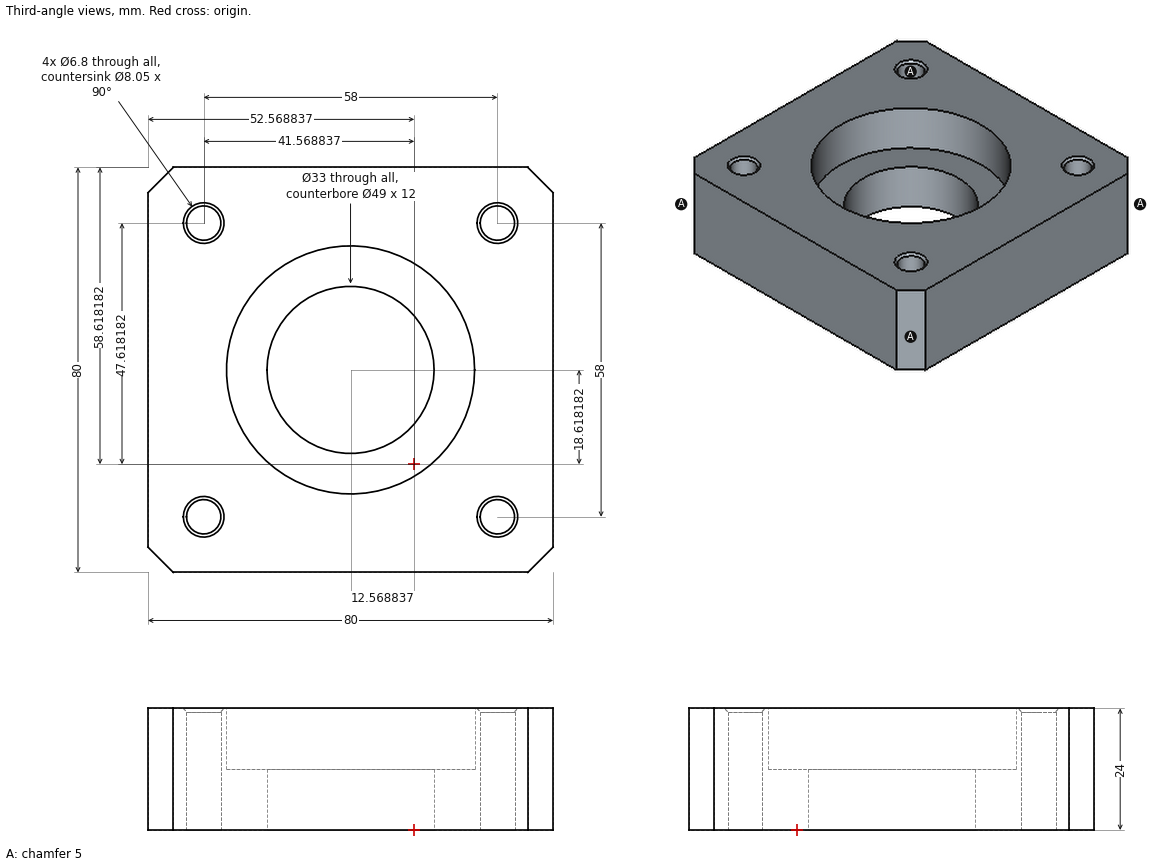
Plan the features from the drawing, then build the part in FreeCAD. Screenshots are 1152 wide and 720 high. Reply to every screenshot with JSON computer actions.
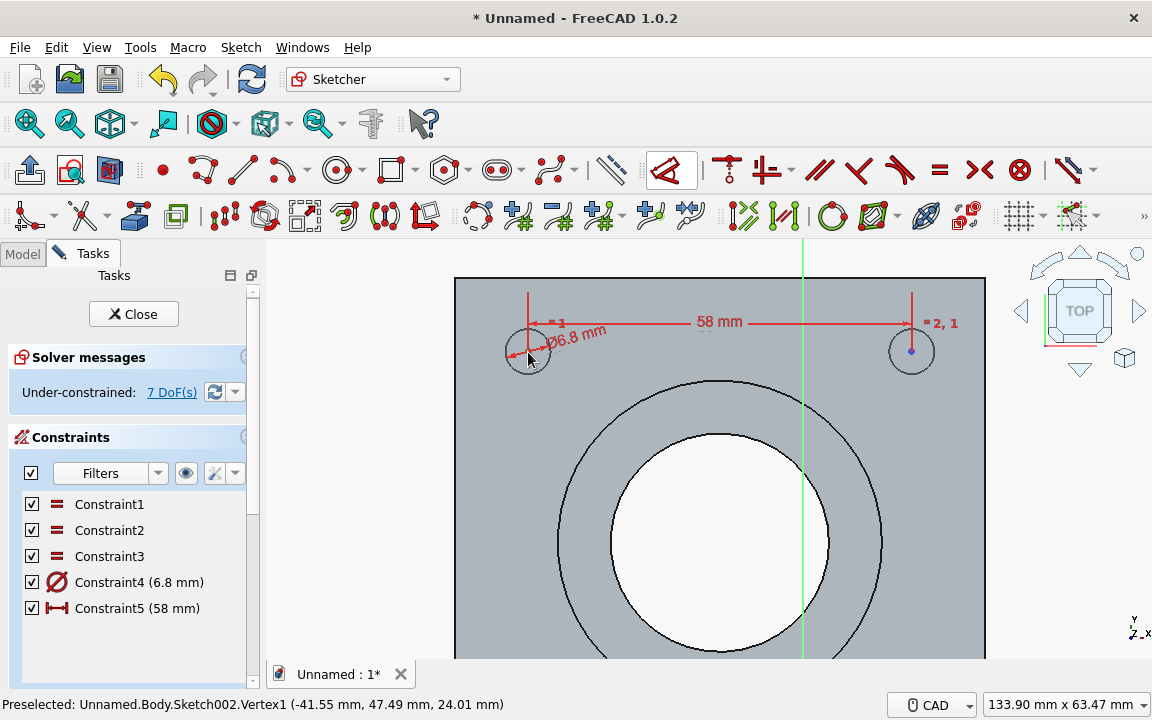
{"action": "scroll", "coordinate": [544, 335], "scroll_direction": "down", "scroll_amount": 3}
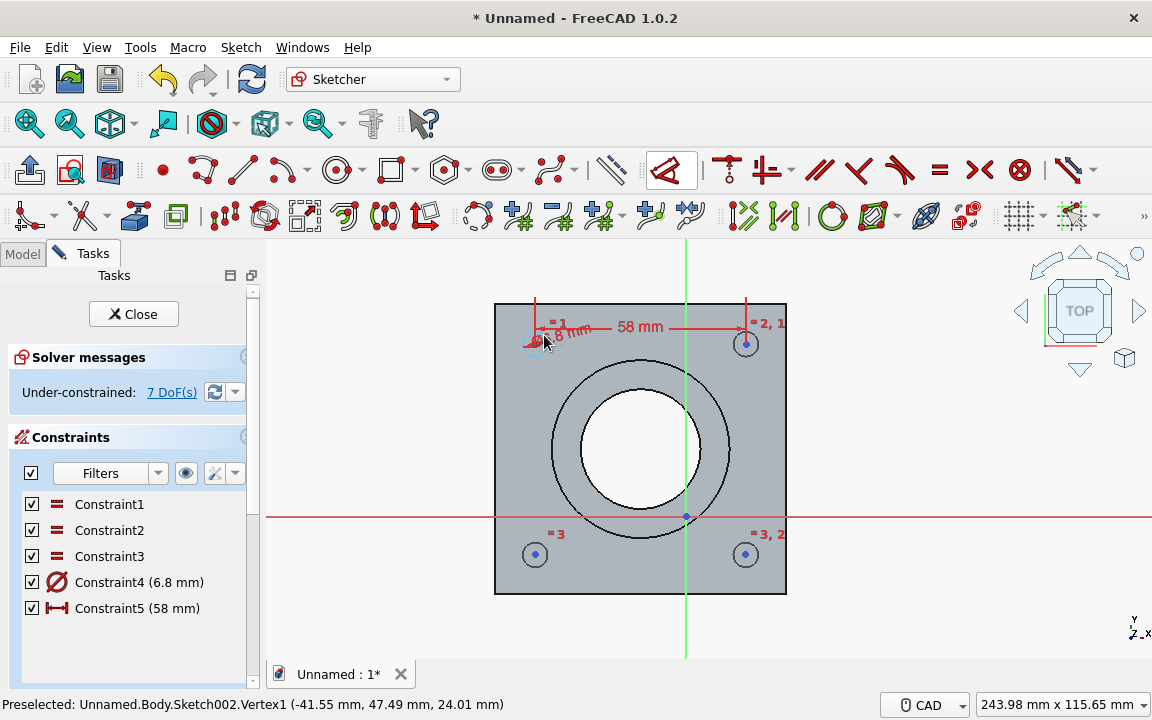
{"action": "left_click", "coordinate": [746, 555]}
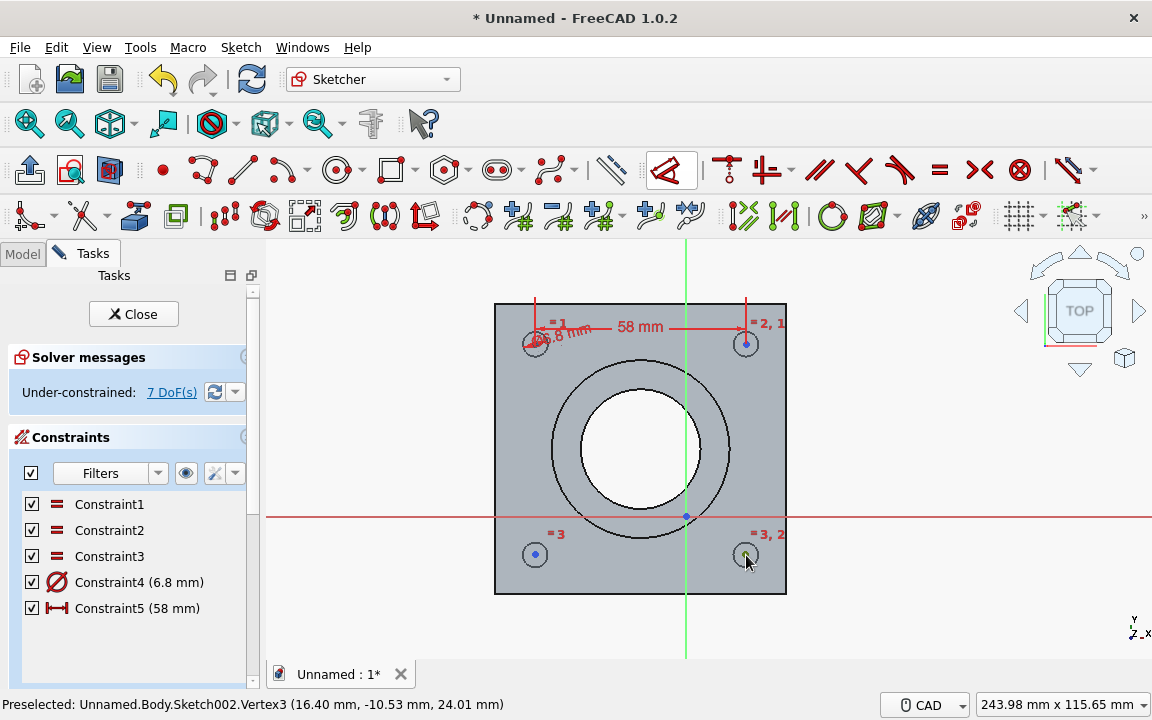
{"action": "key", "text": "l"}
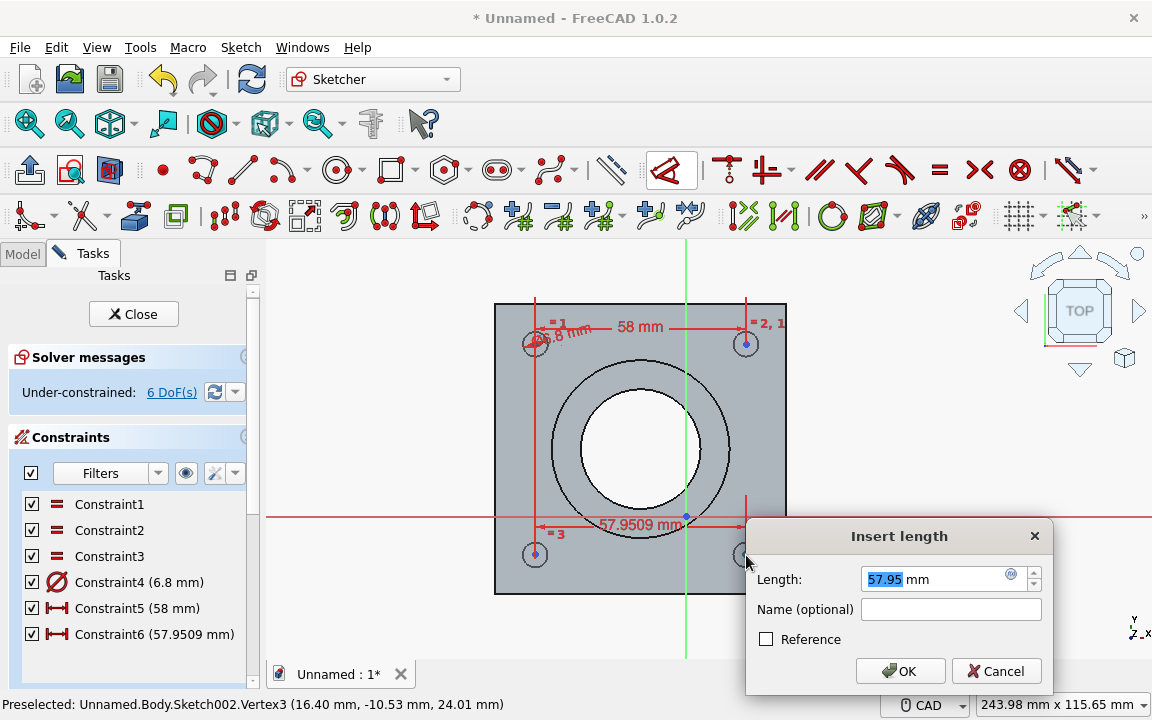
{"action": "type", "text": "58"}
{"action": "key", "text": "Return"}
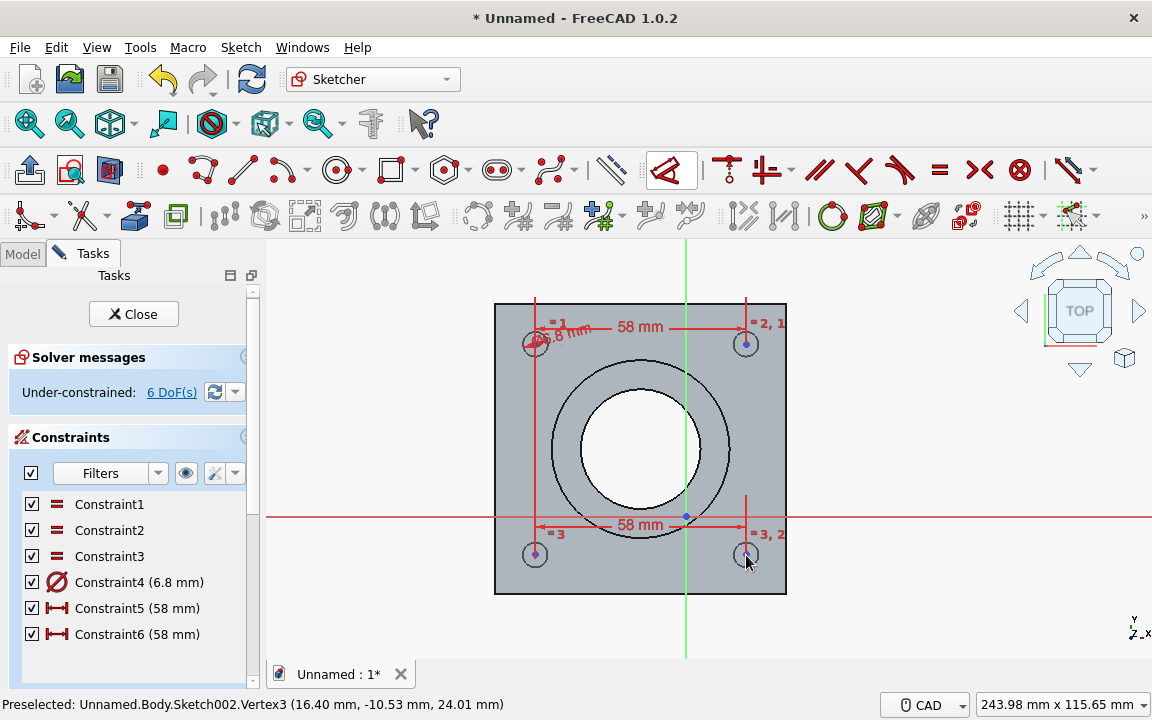
{"action": "left_click", "coordinate": [746, 344]}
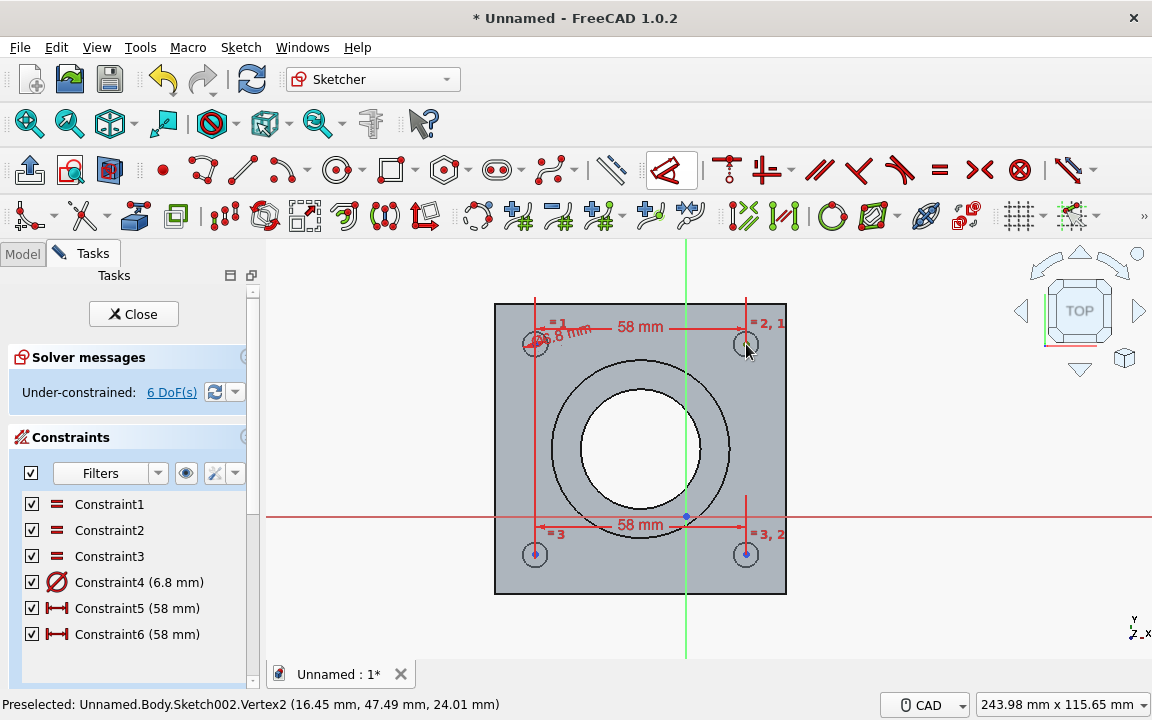
{"action": "left_click", "coordinate": [746, 555]}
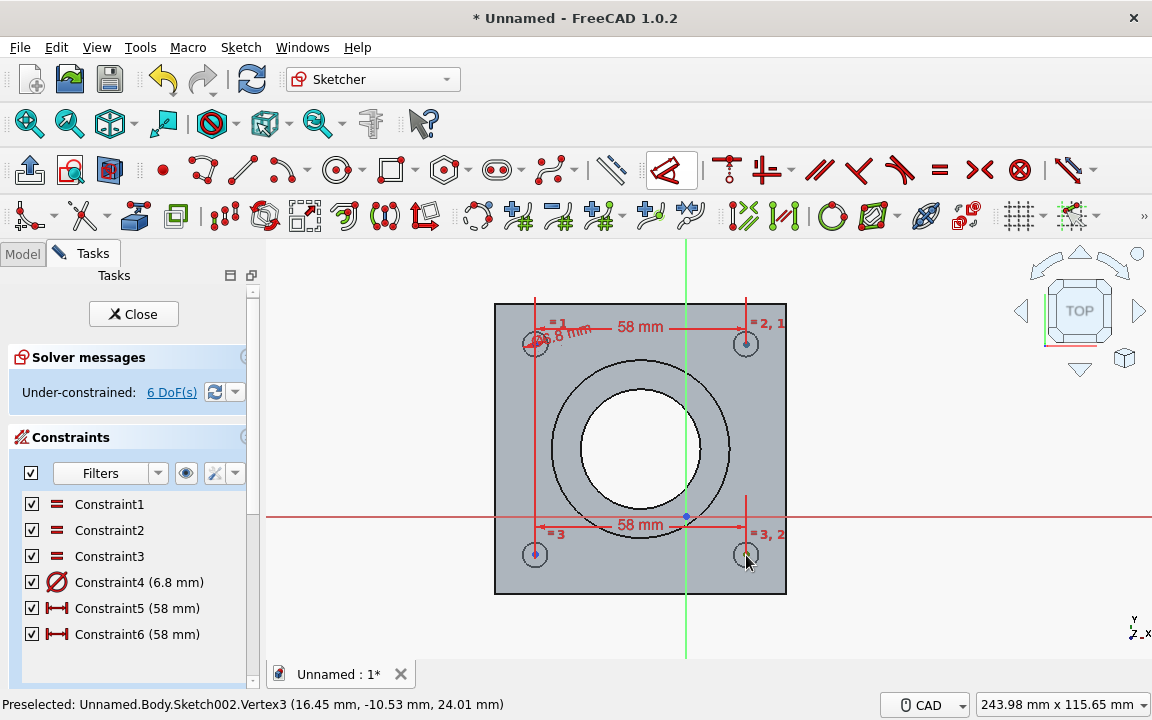
{"action": "left_click", "coordinate": [692, 170]}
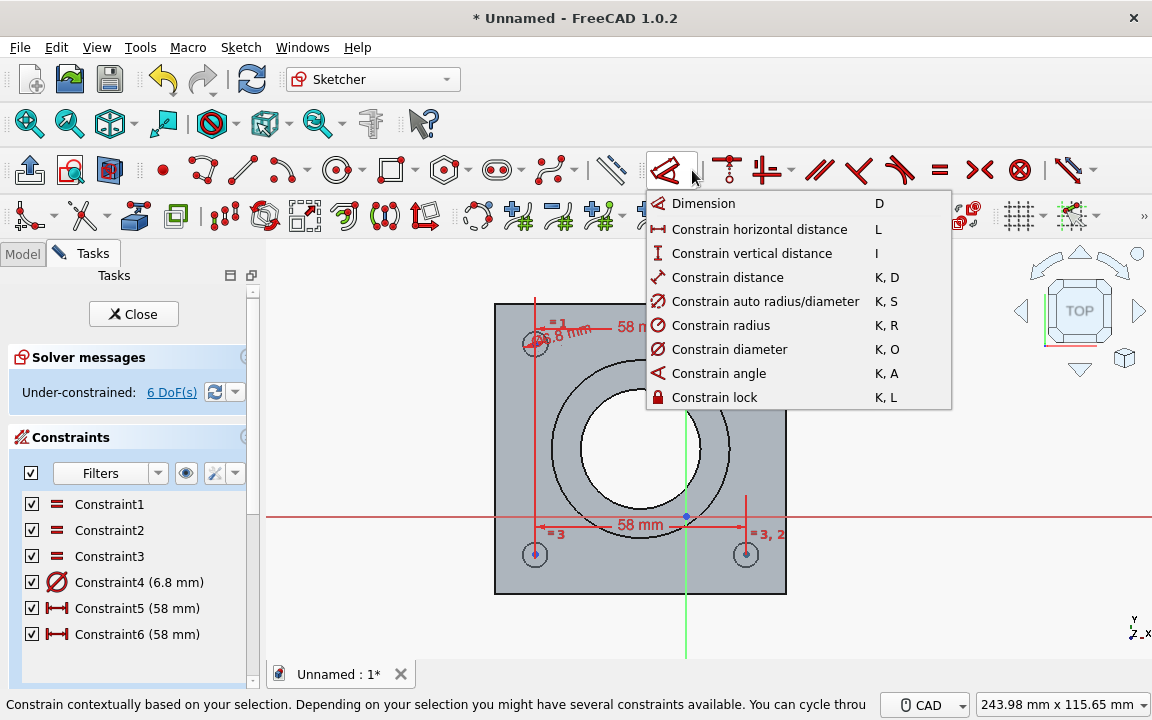
{"action": "left_click", "coordinate": [799, 253]}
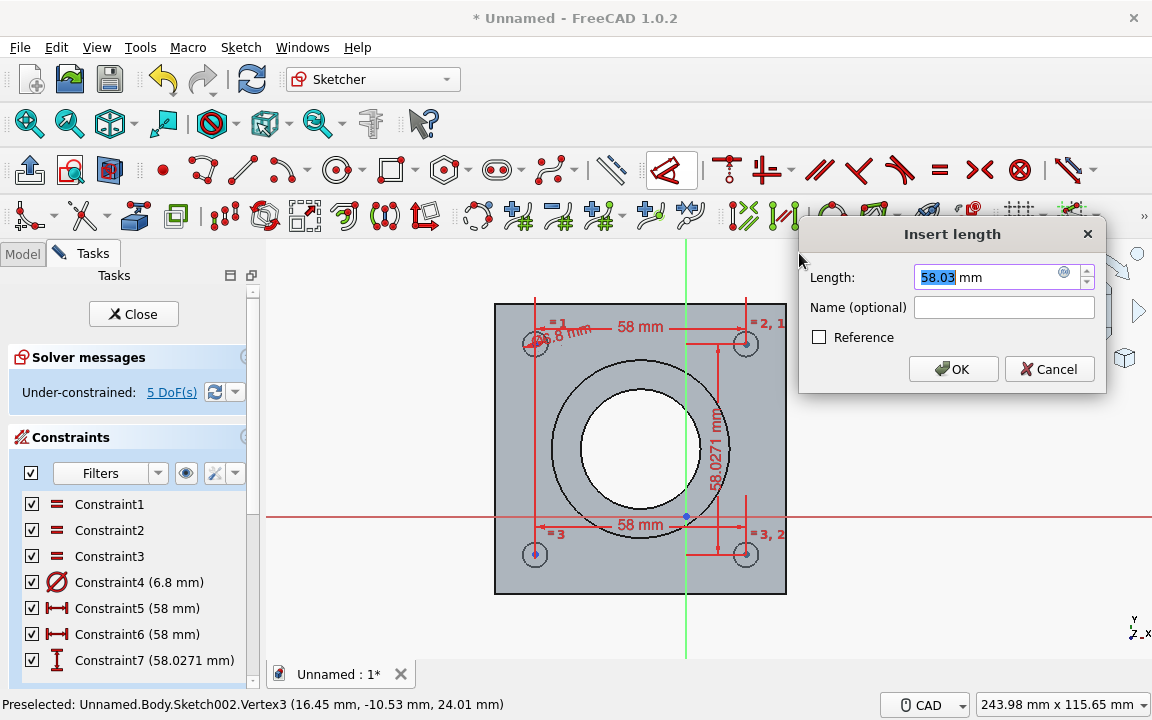
{"action": "type", "text": "58"}
{"action": "key", "text": "Return"}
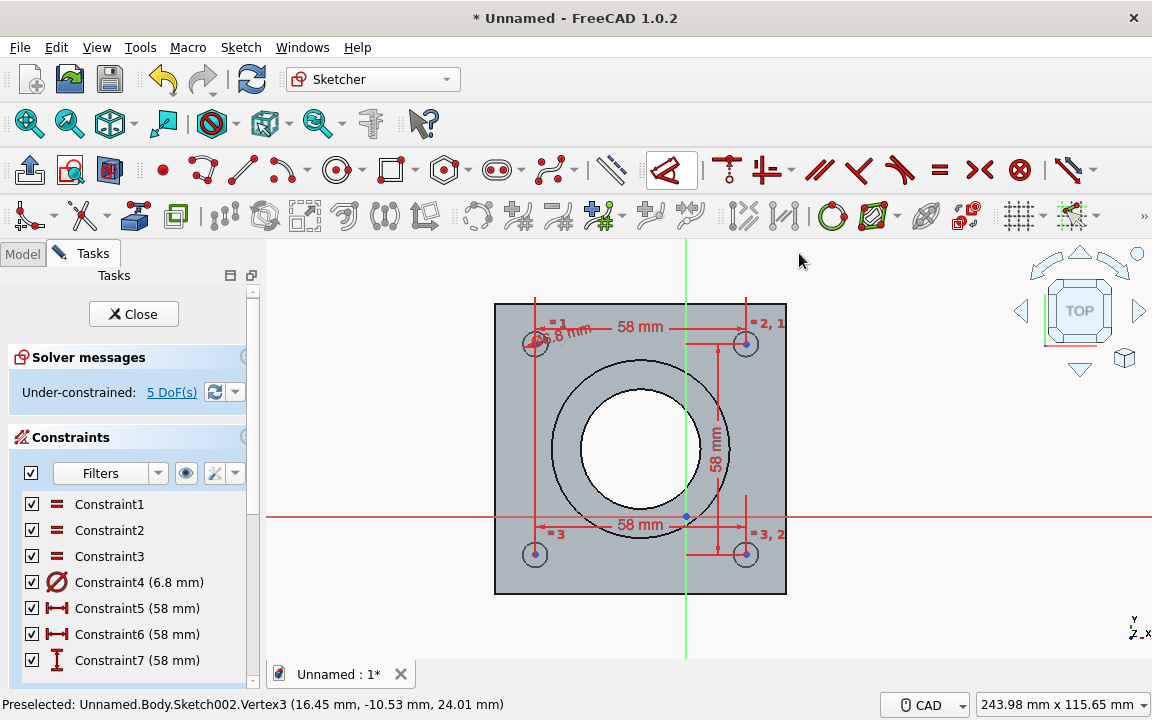
{"action": "left_click", "coordinate": [535, 344]}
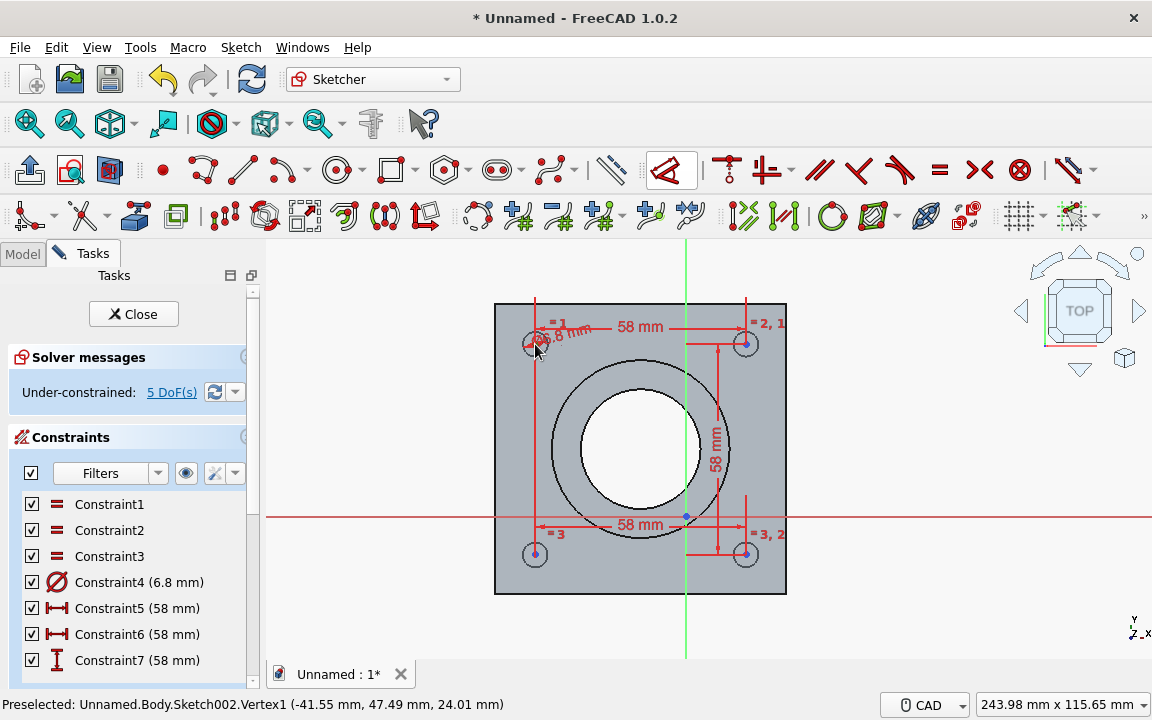
{"action": "left_click", "coordinate": [746, 555]}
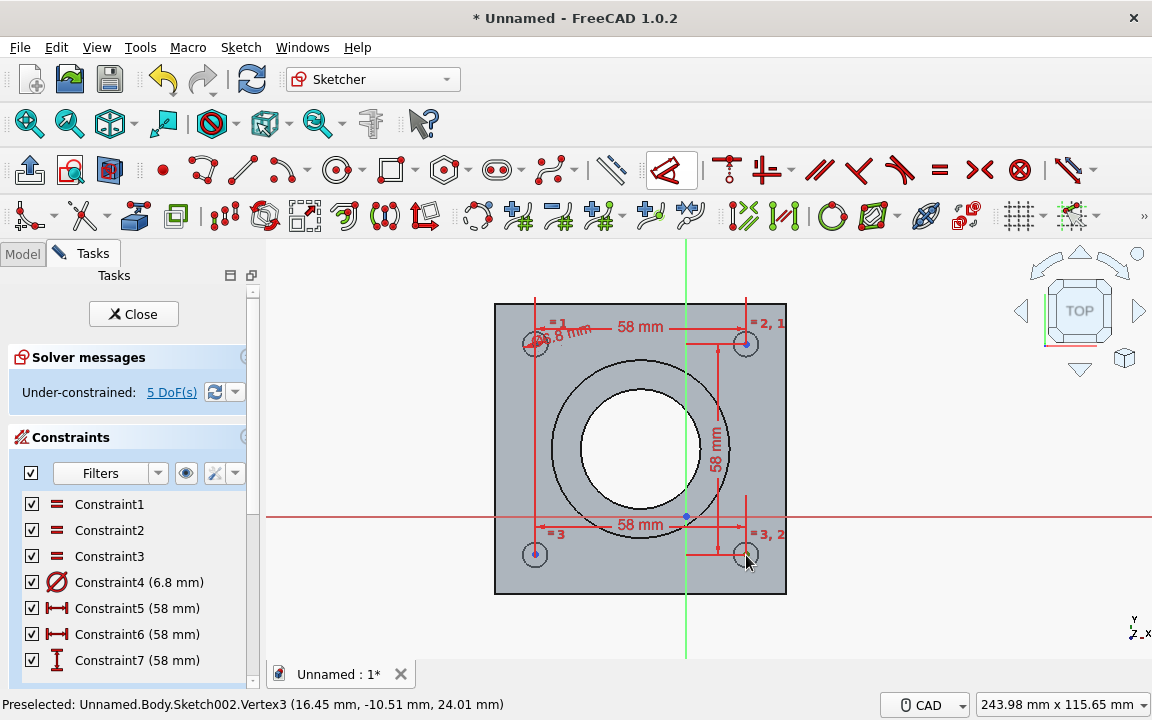
{"action": "left_click", "coordinate": [692, 170]}